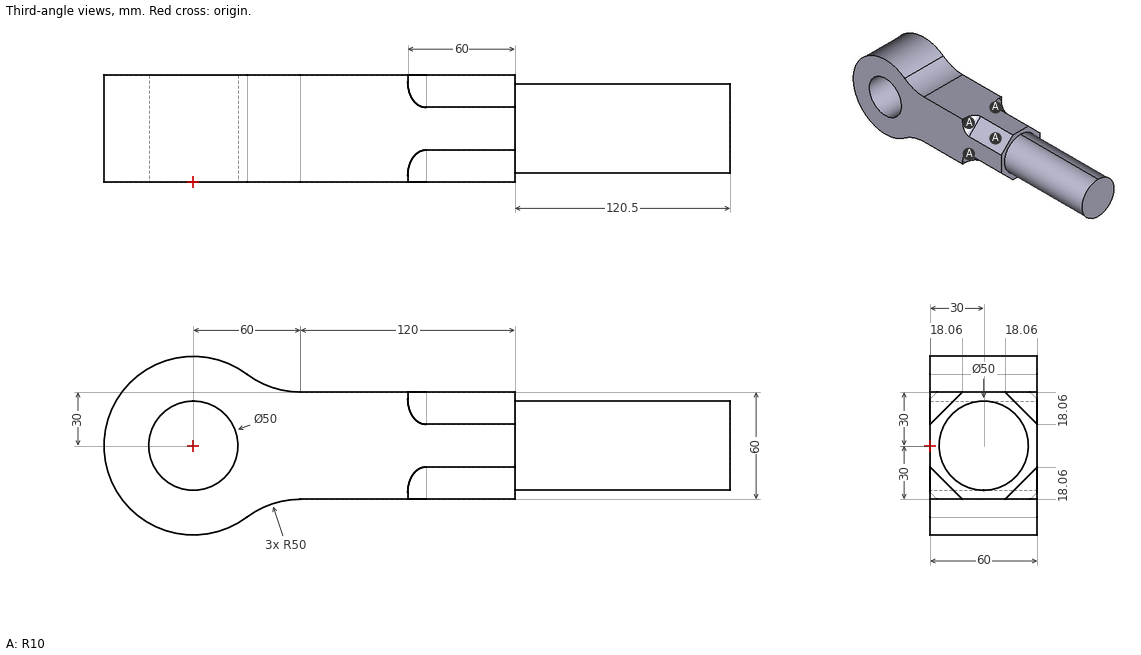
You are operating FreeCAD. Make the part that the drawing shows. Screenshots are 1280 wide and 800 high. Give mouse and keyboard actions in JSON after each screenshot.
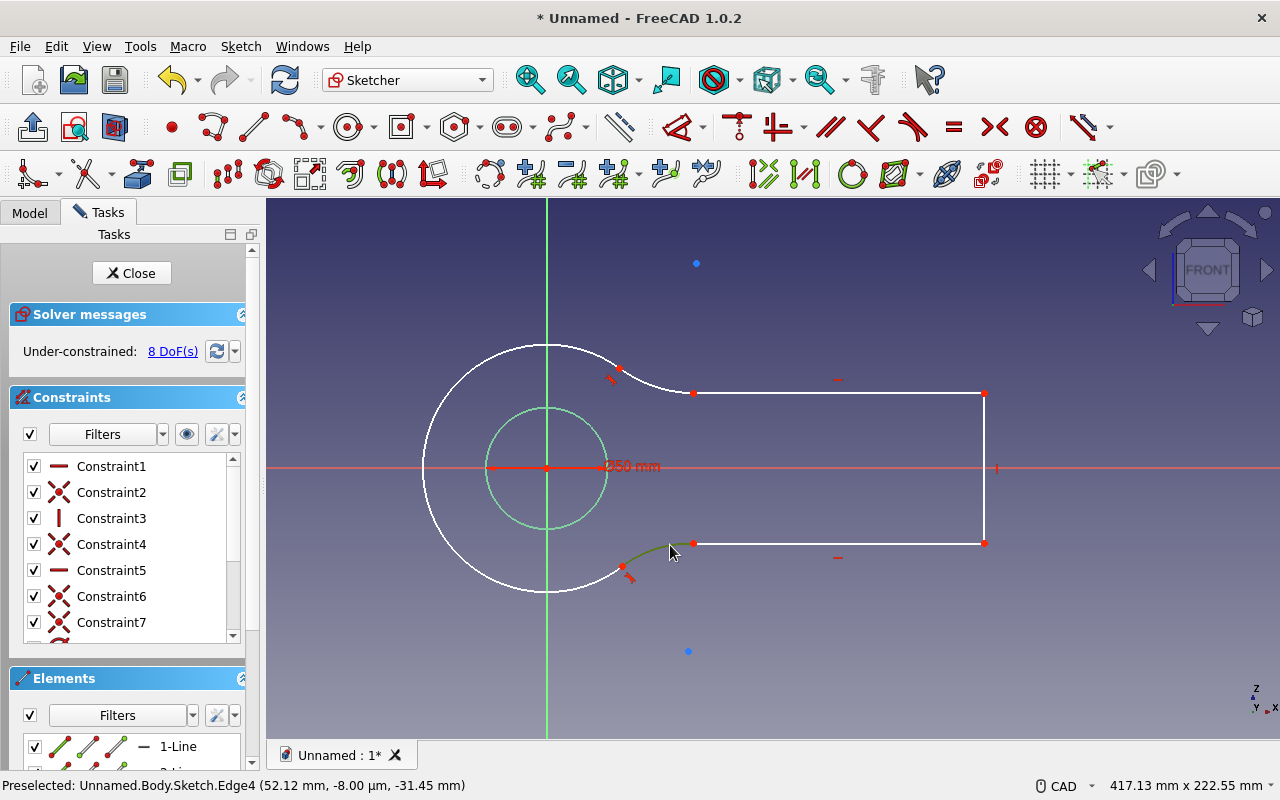
{"action": "left_click", "coordinate": [467, 374]}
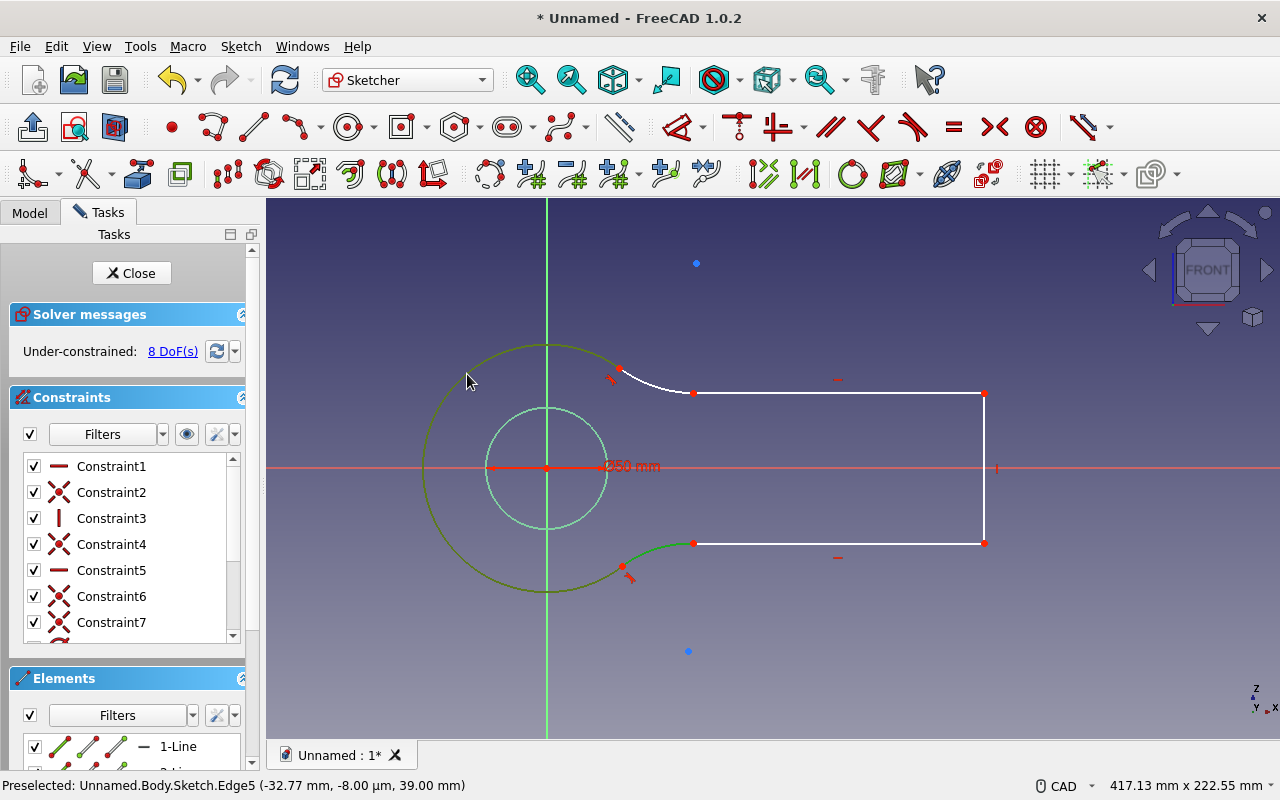
{"action": "left_click", "coordinate": [640, 380]}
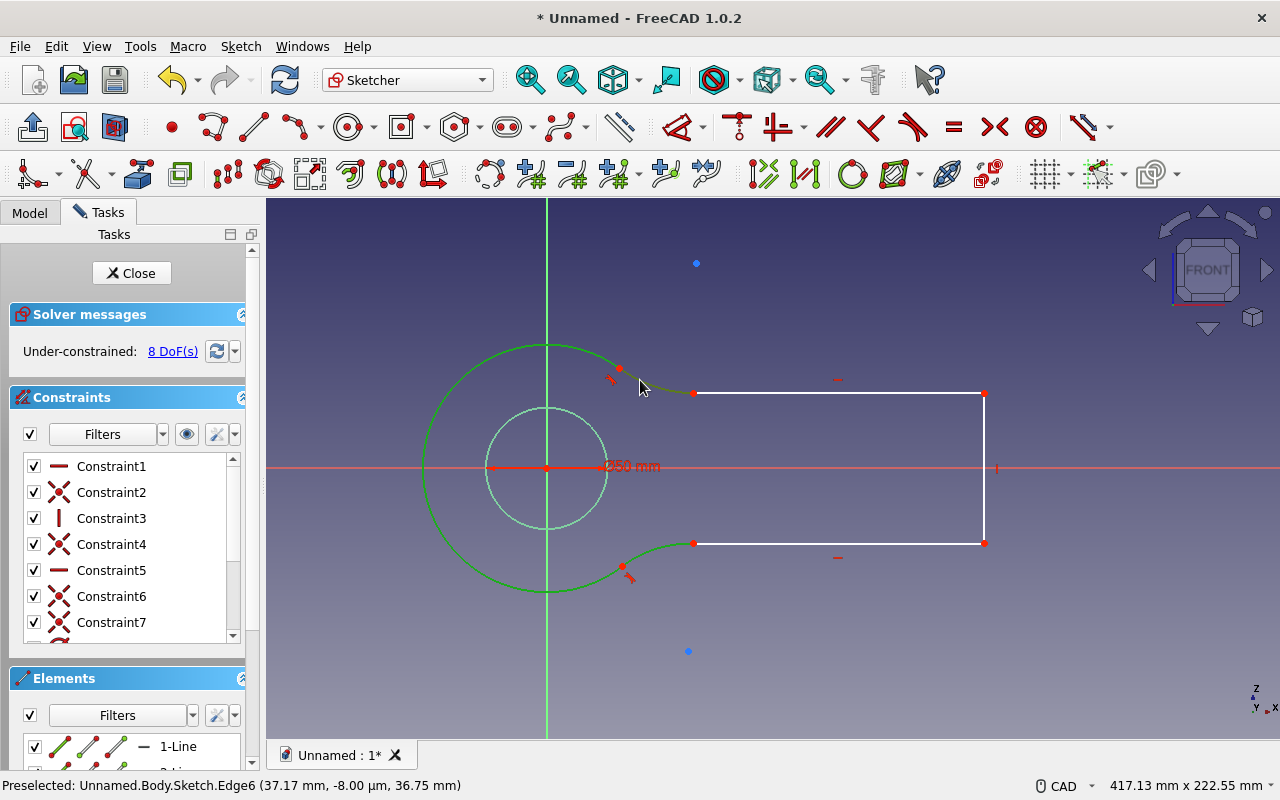
{"action": "key", "text": "e"}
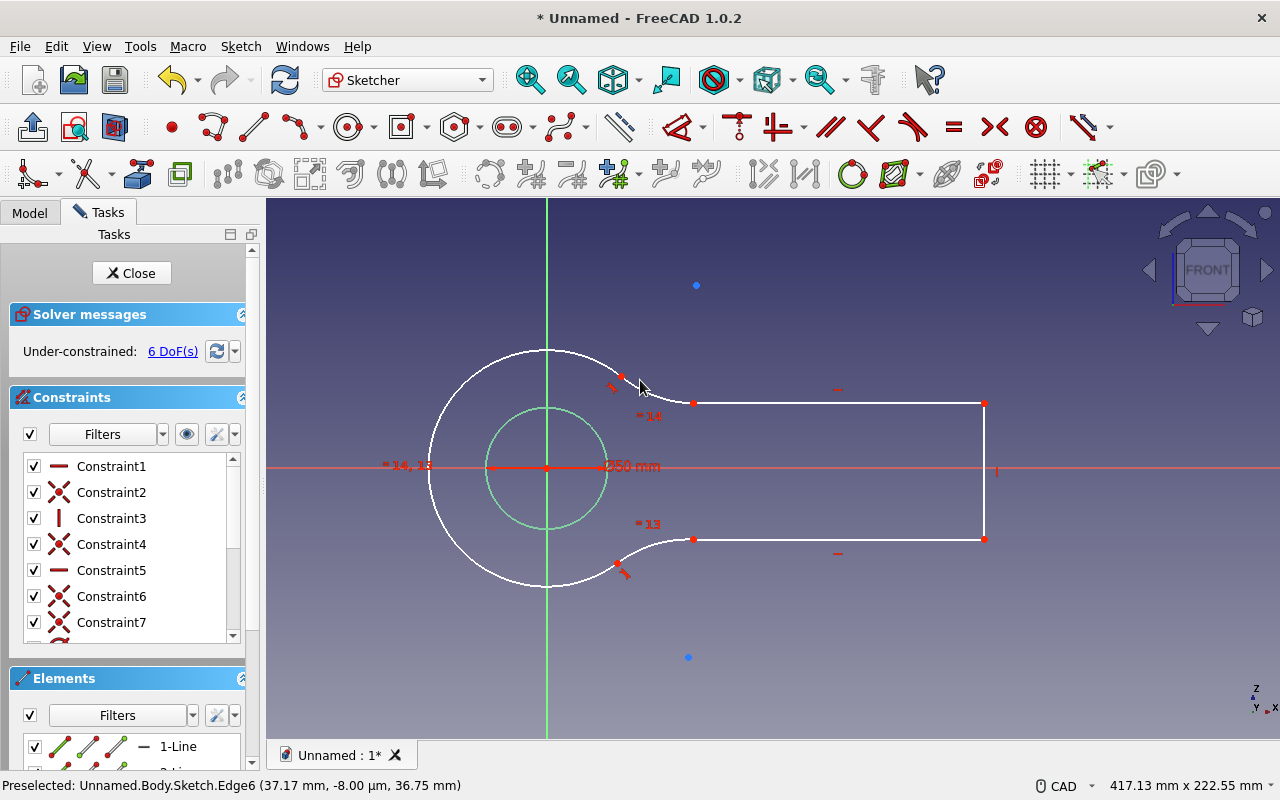
{"action": "key", "text": "d"}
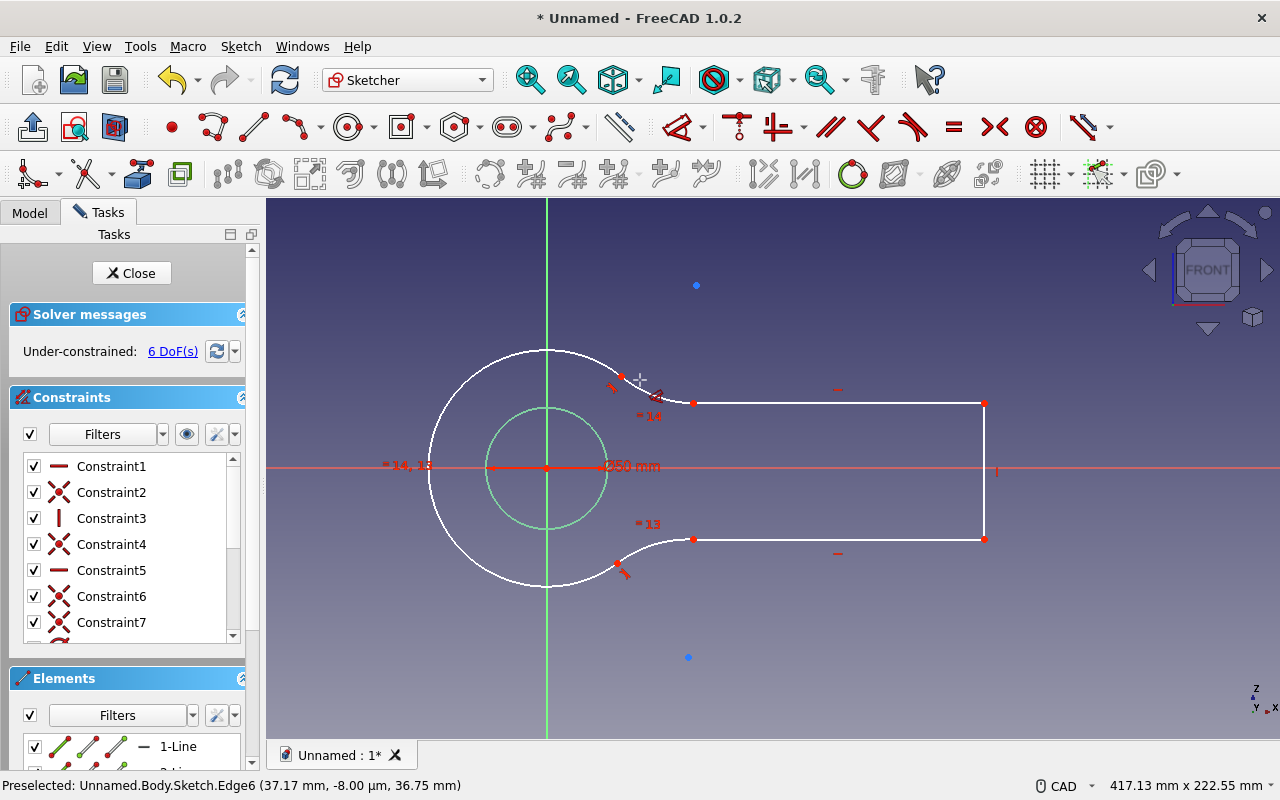
{"action": "left_click", "coordinate": [669, 541]}
{"action": "left_click", "coordinate": [664, 509]}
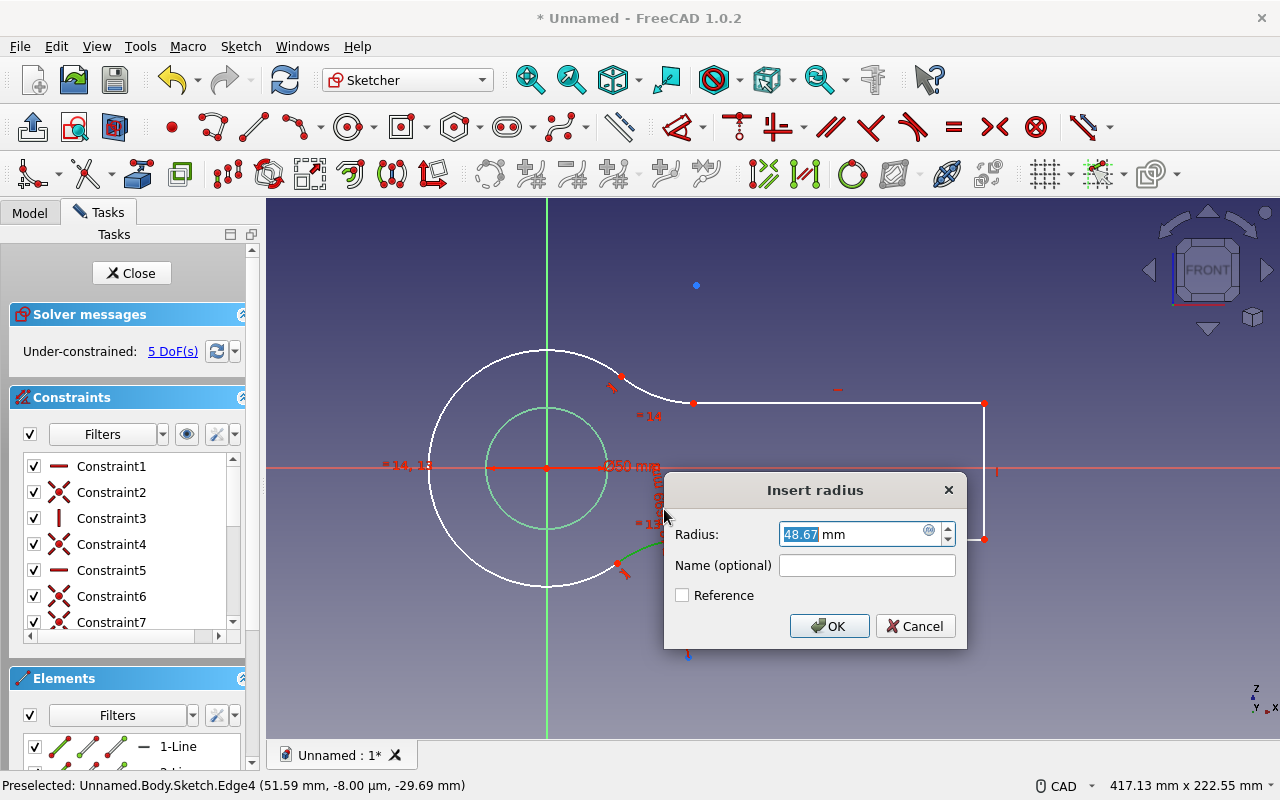
{"action": "type", "text": "50"}
{"action": "key", "text": "Return"}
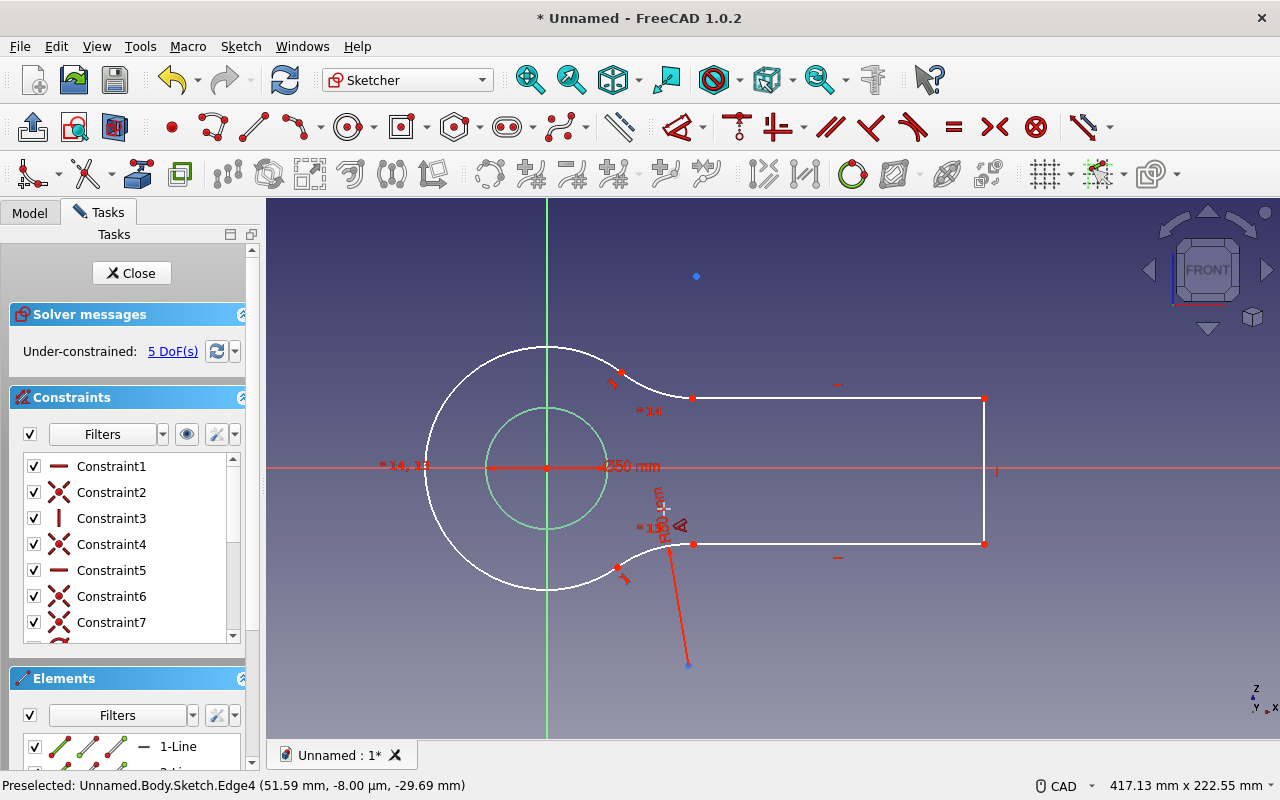
{"action": "left_click", "coordinate": [984, 442]}
{"action": "left_click", "coordinate": [1018, 438]}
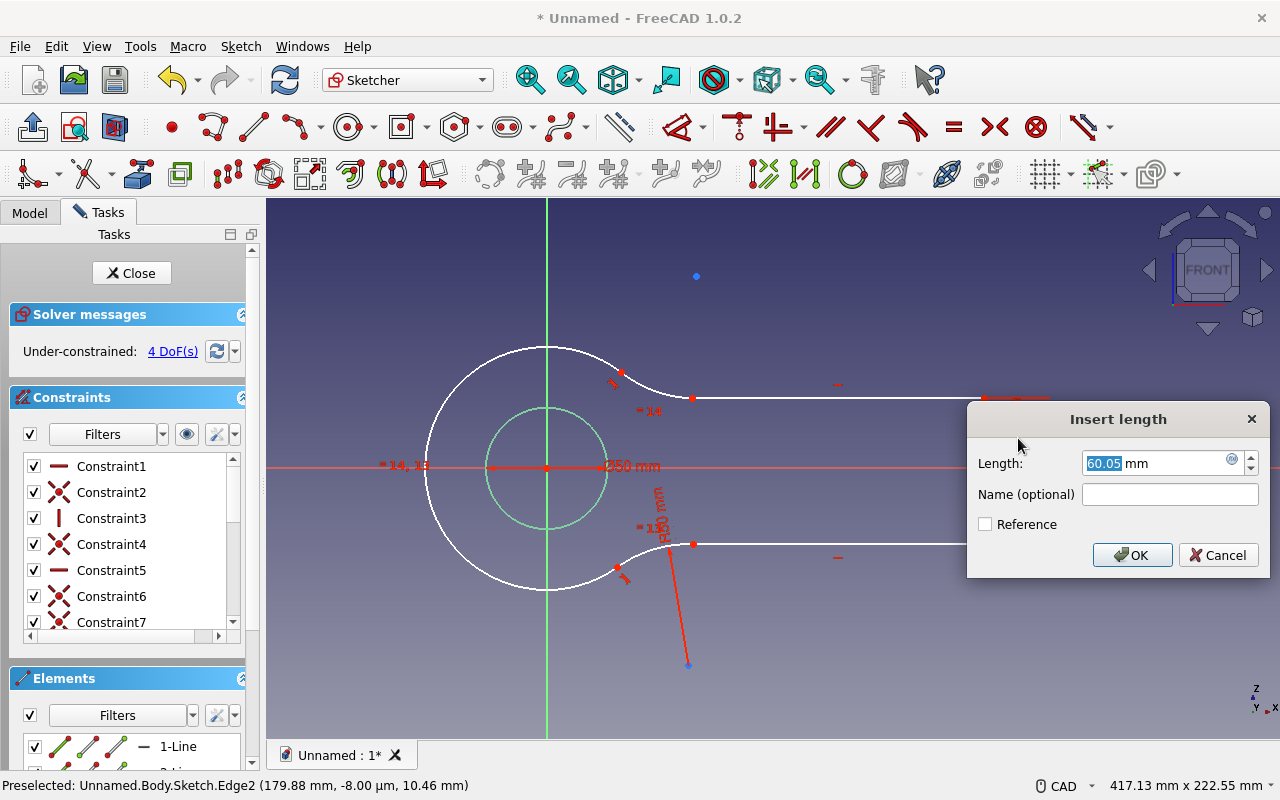
{"action": "type", "text": "60"}
{"action": "key", "text": "Return"}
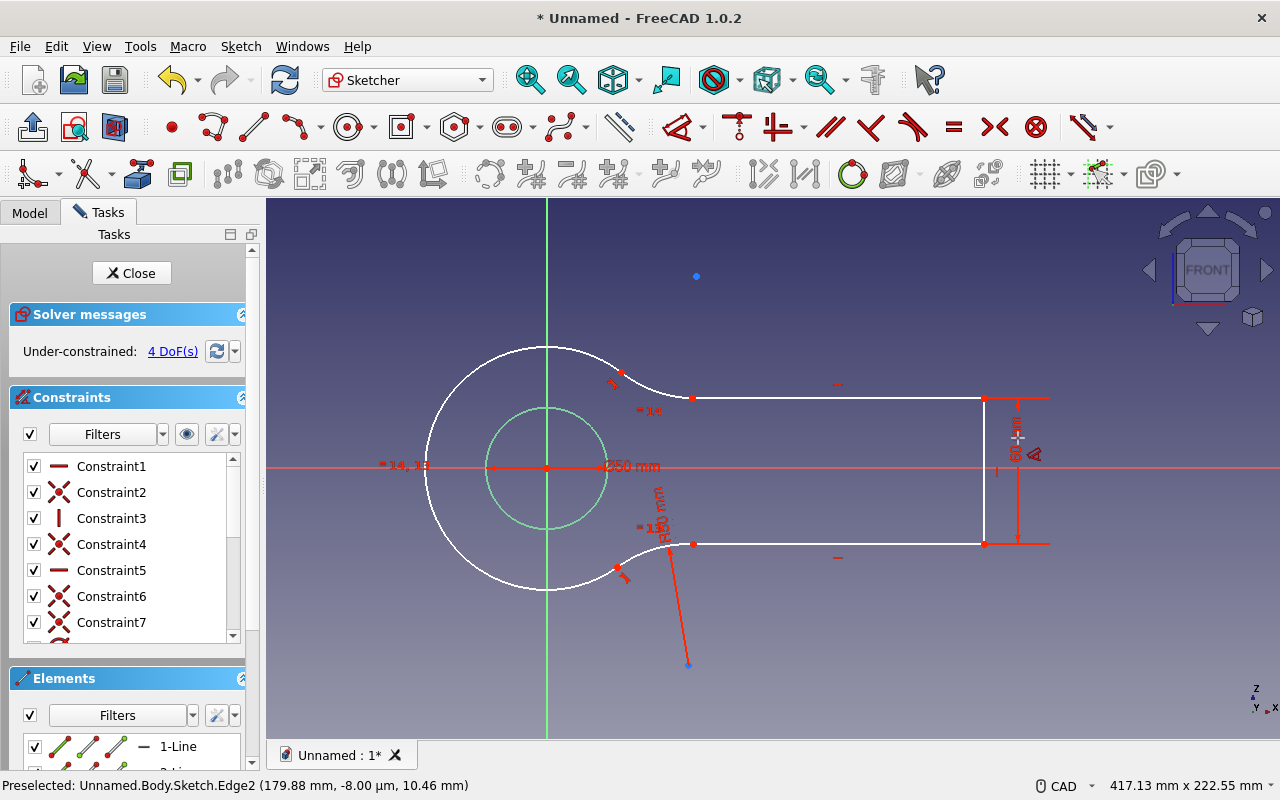
{"action": "left_click", "coordinate": [780, 398]}
{"action": "left_click", "coordinate": [838, 364]}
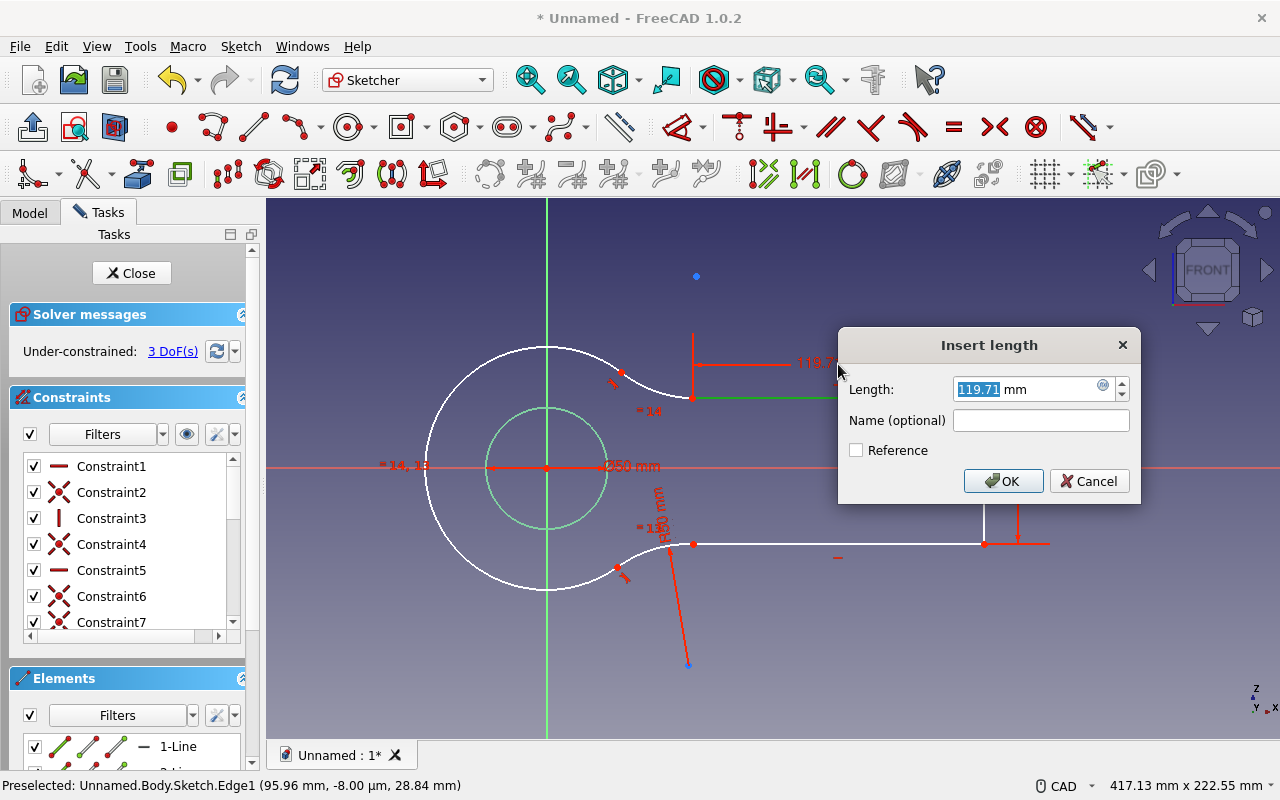
{"action": "type", "text": "120"}
{"action": "key", "text": "Return"}